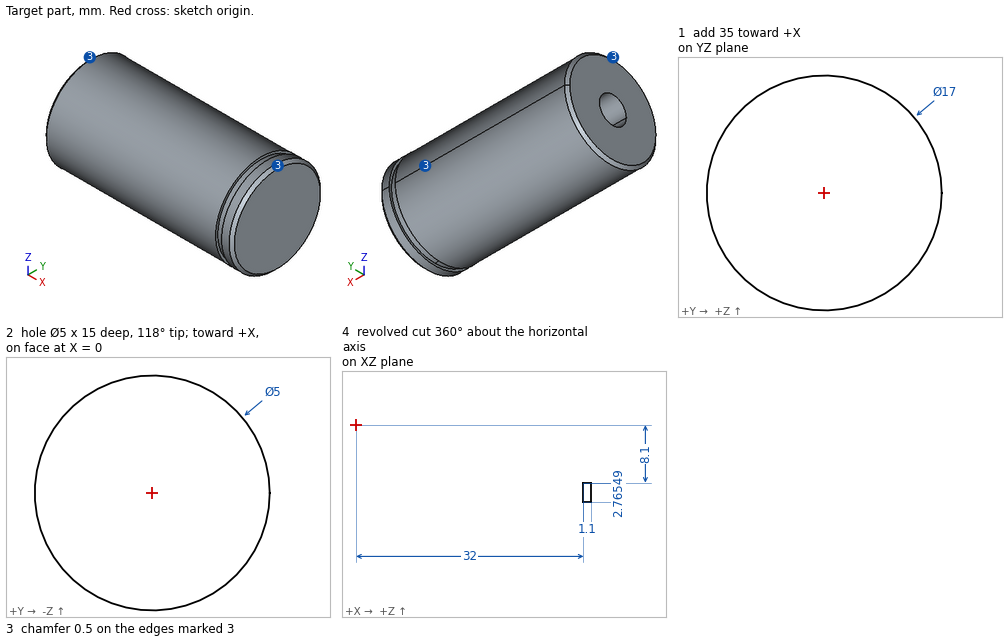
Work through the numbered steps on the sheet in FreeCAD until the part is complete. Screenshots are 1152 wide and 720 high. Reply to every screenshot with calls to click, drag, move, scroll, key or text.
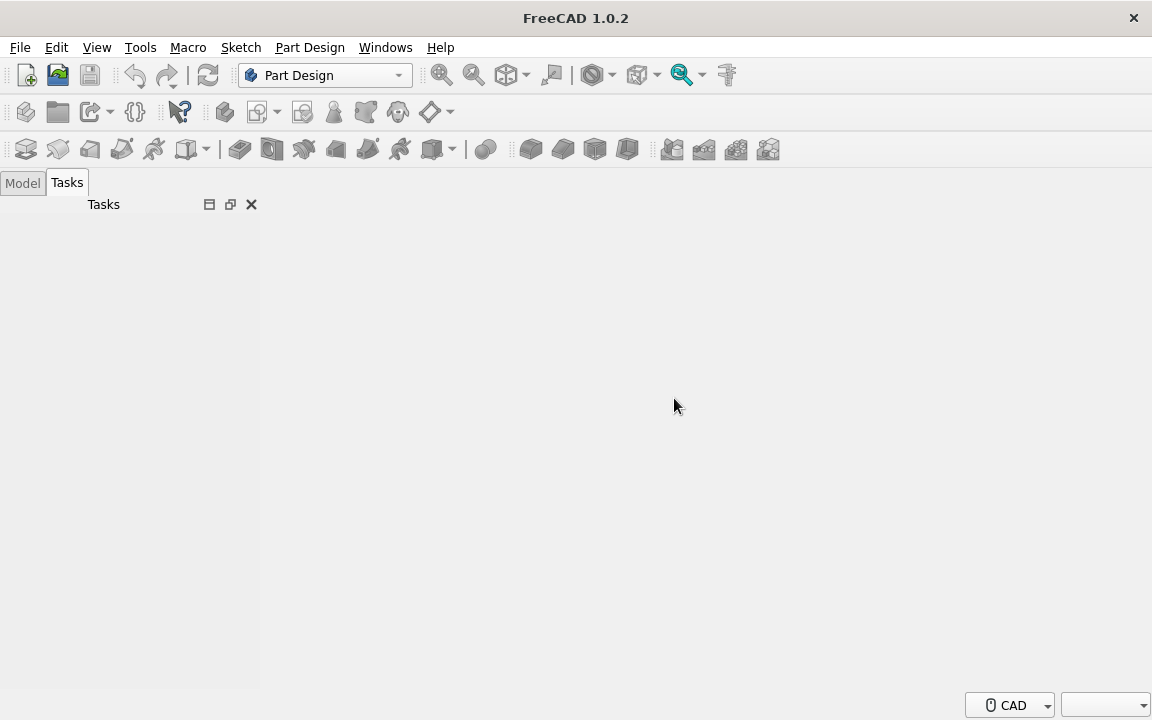
click(26, 76)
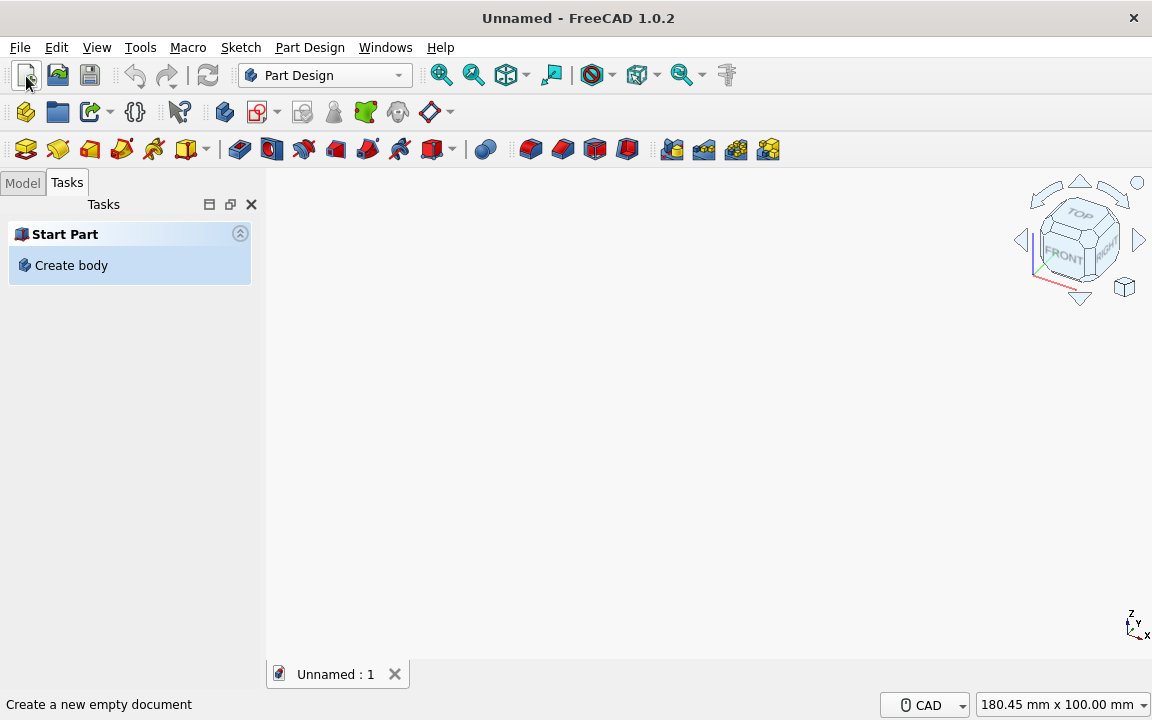
click(258, 112)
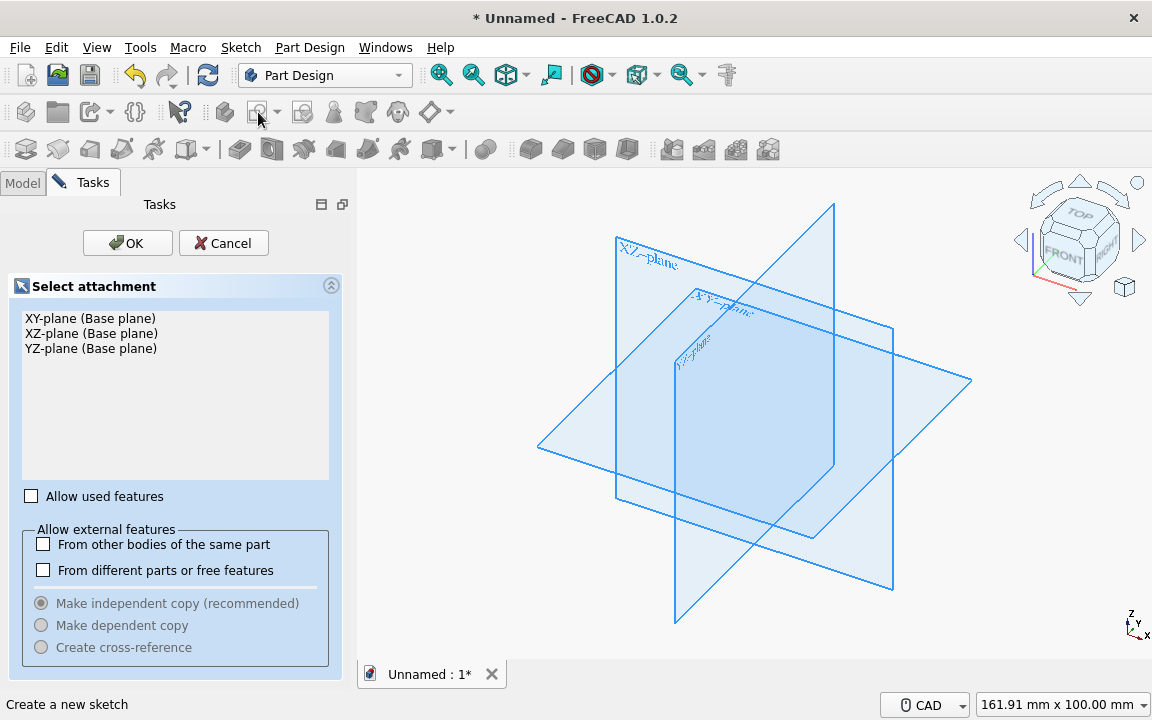
click(82, 348)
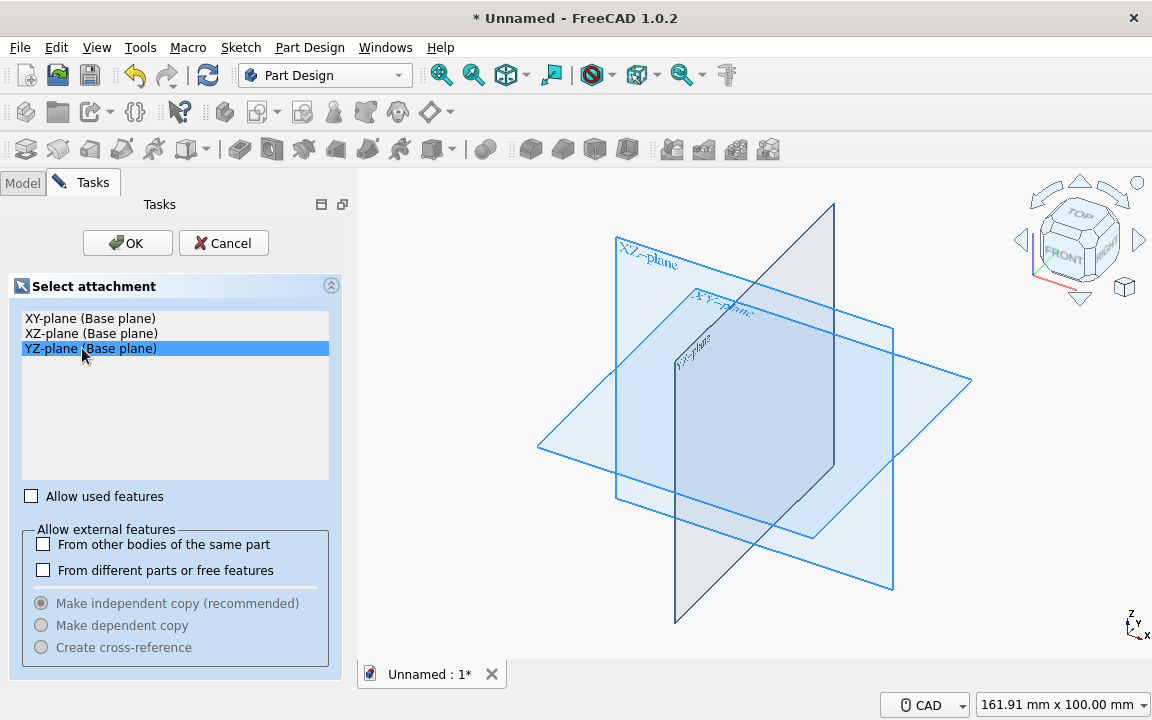
click(128, 243)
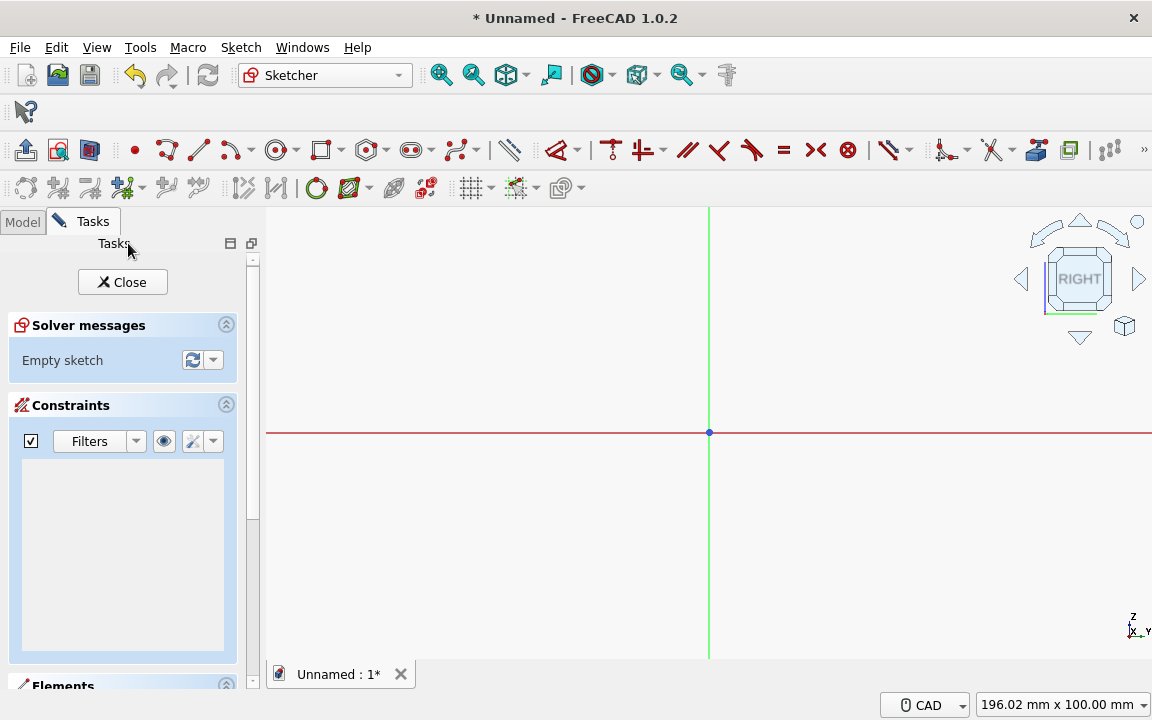
scroll(739, 433, up, 6)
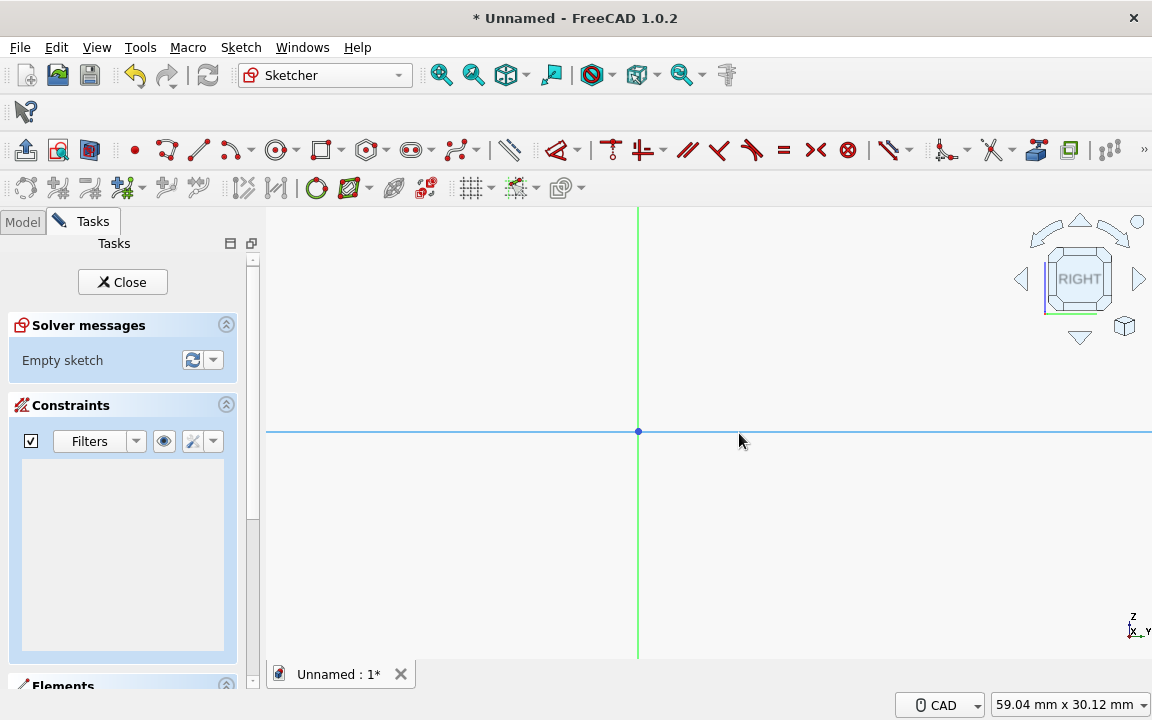
click(276, 150)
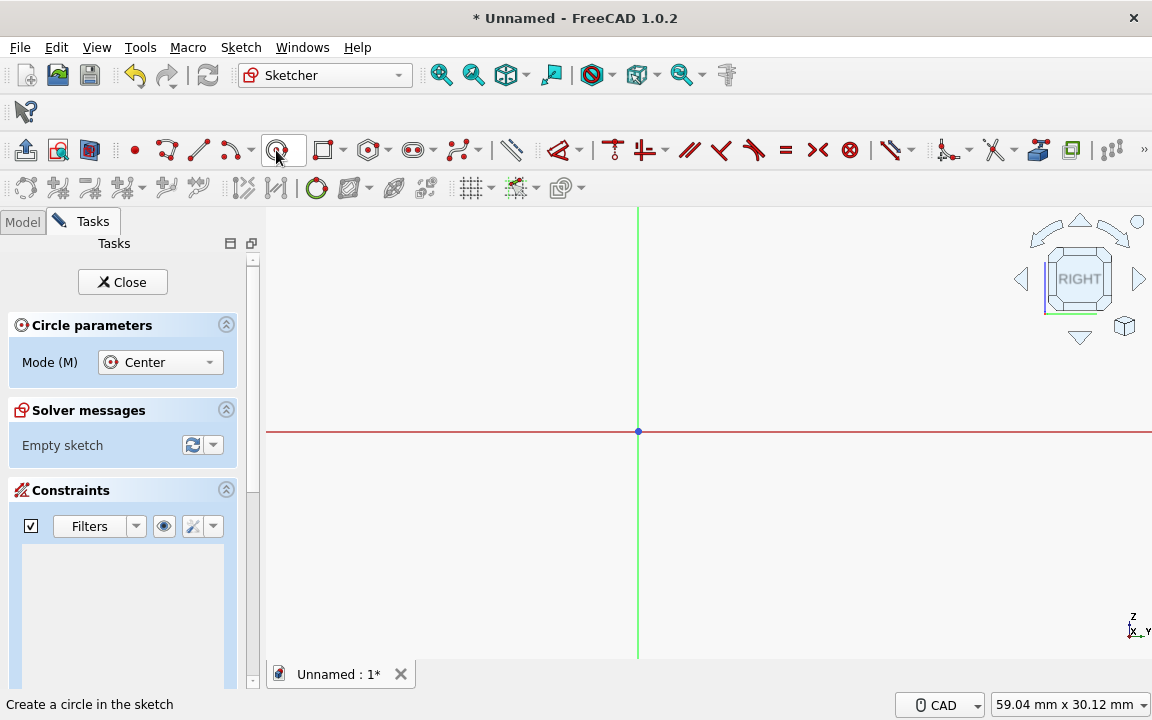
click(638, 432)
click(728, 342)
key(Escape)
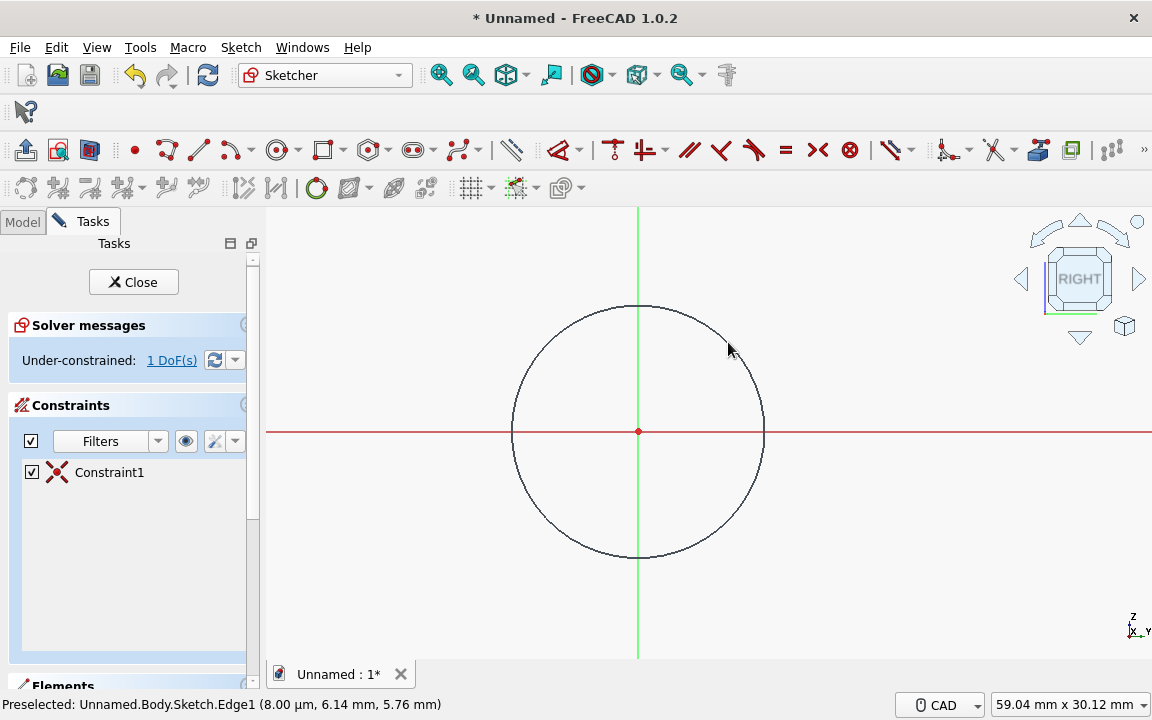
click(558, 150)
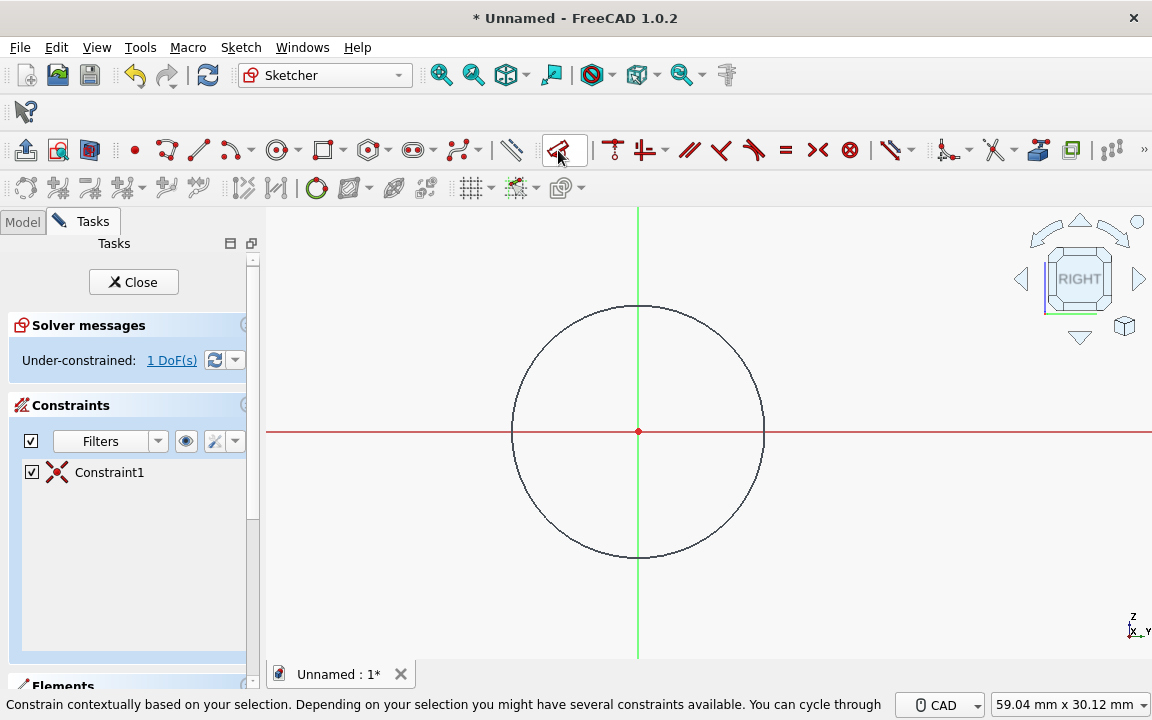
click(727, 342)
click(750, 319)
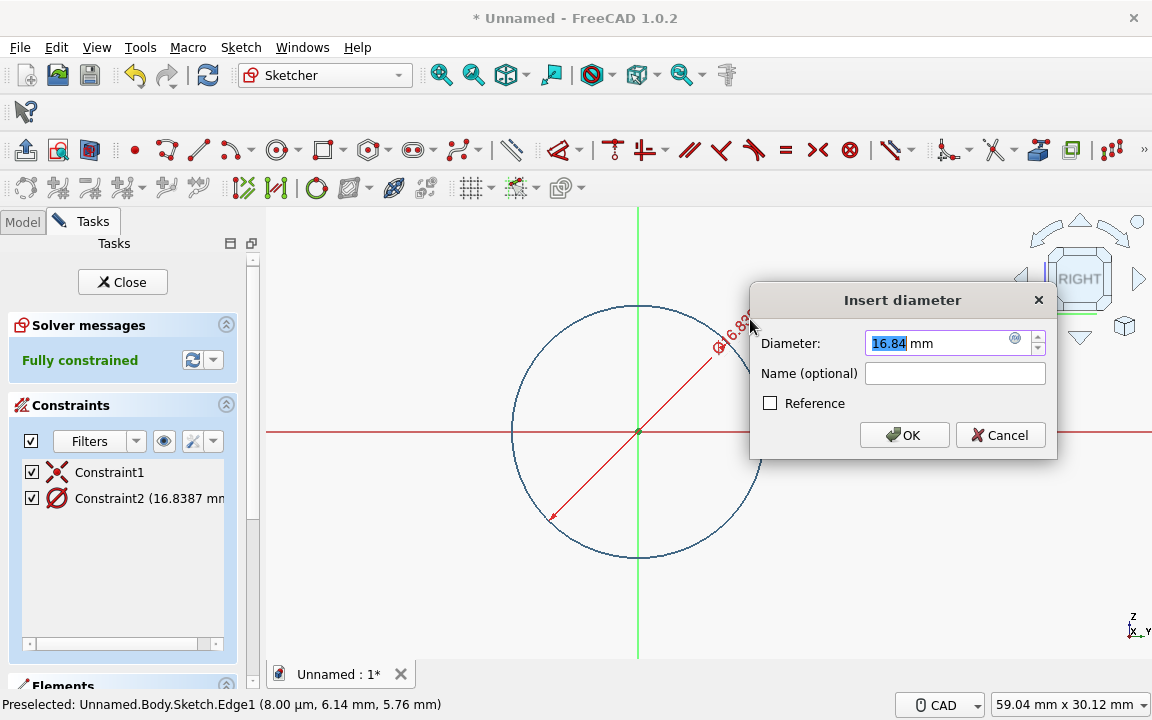
text(17)
key(Return)
key(Escape)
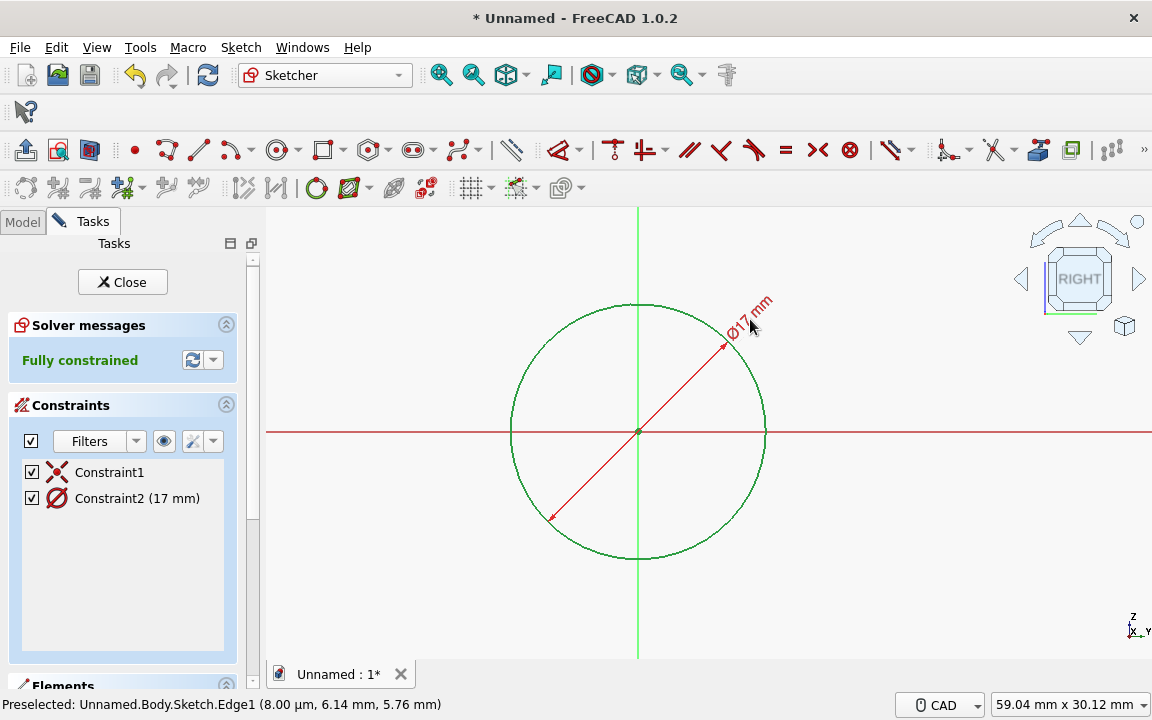
click(123, 282)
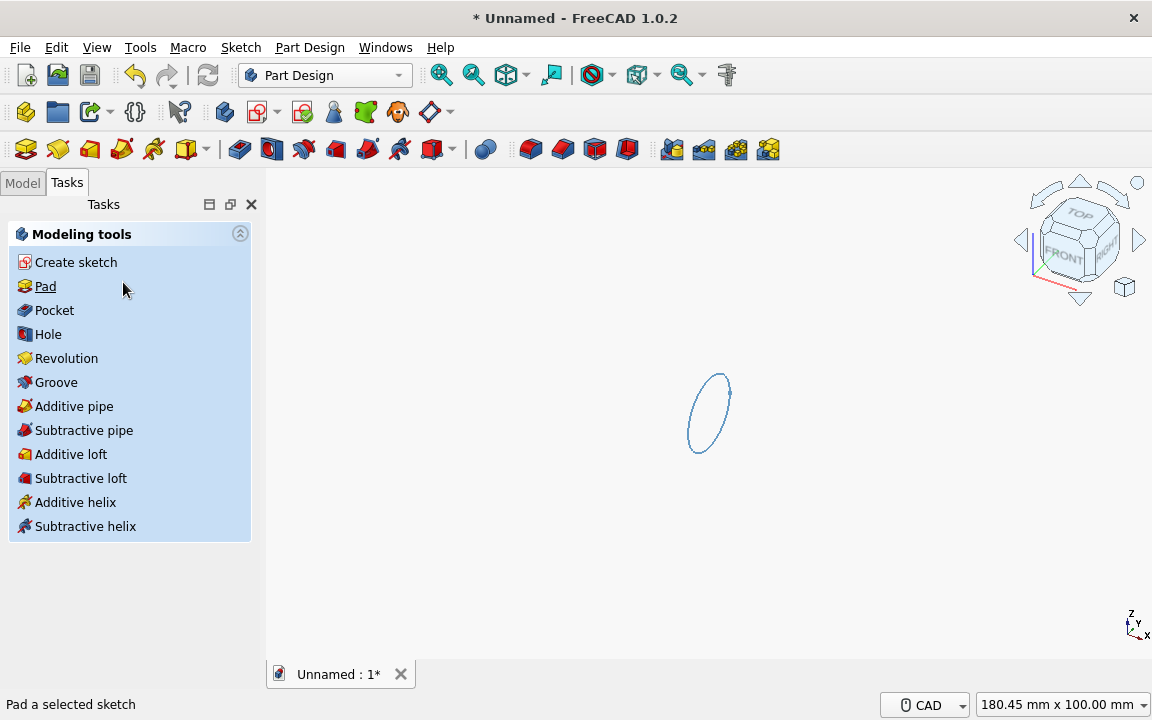
click(26, 150)